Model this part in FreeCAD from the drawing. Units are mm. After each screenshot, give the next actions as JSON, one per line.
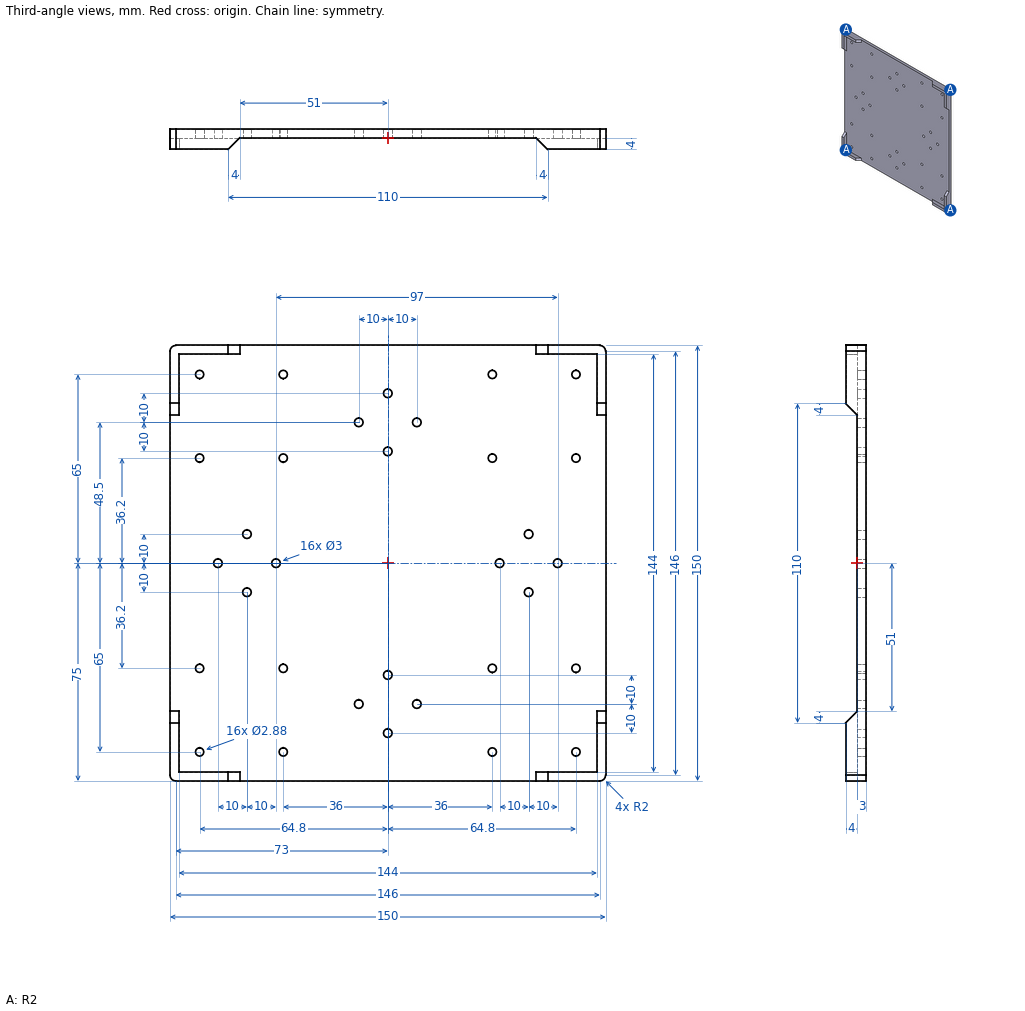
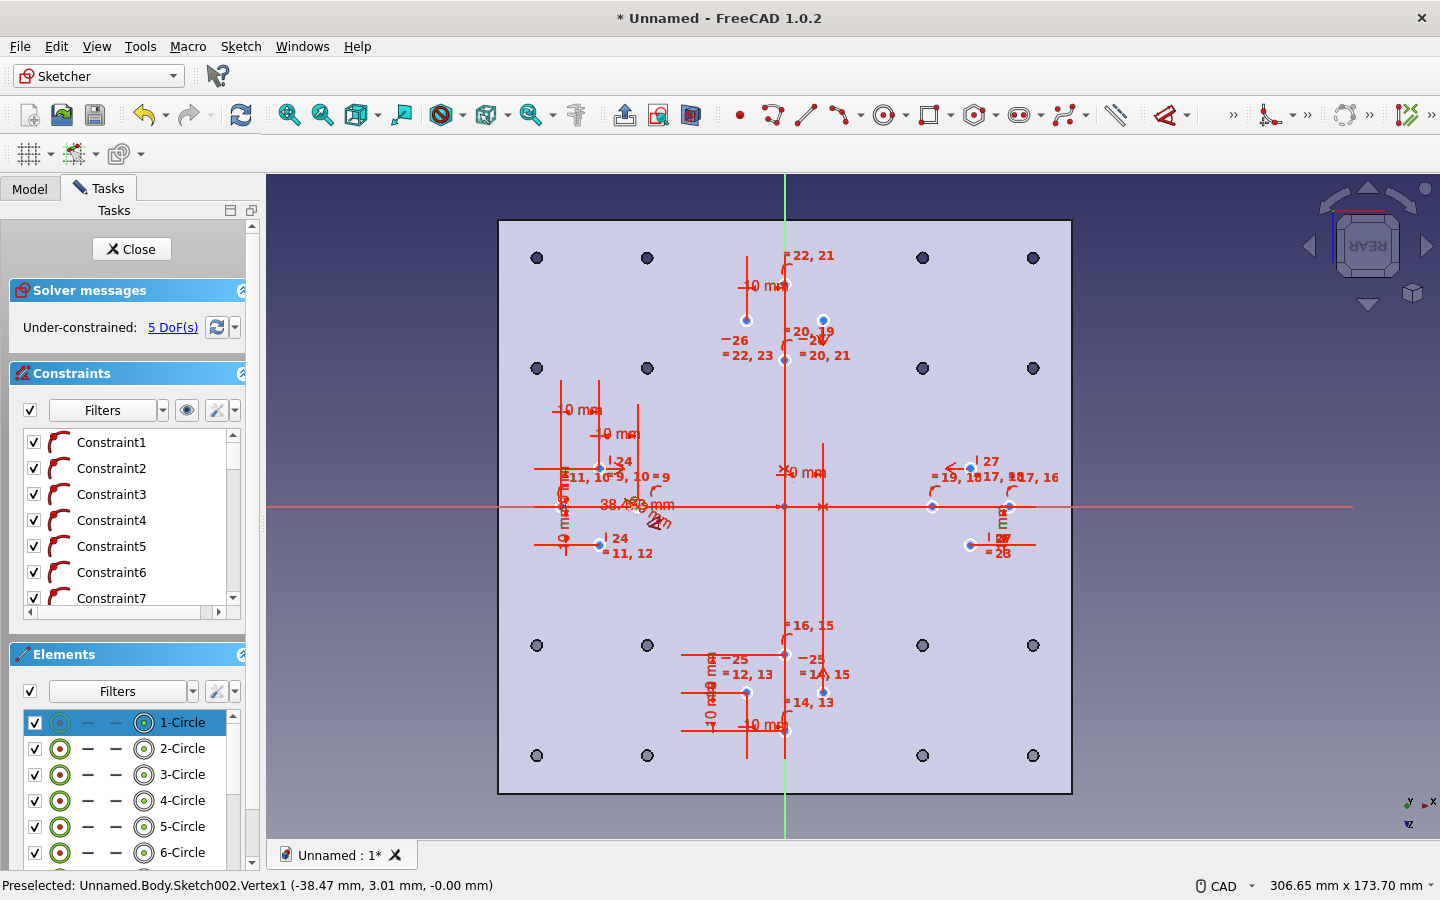
{"action": "left_click", "coordinate": [1009, 507]}
{"action": "left_click", "coordinate": [823, 541]}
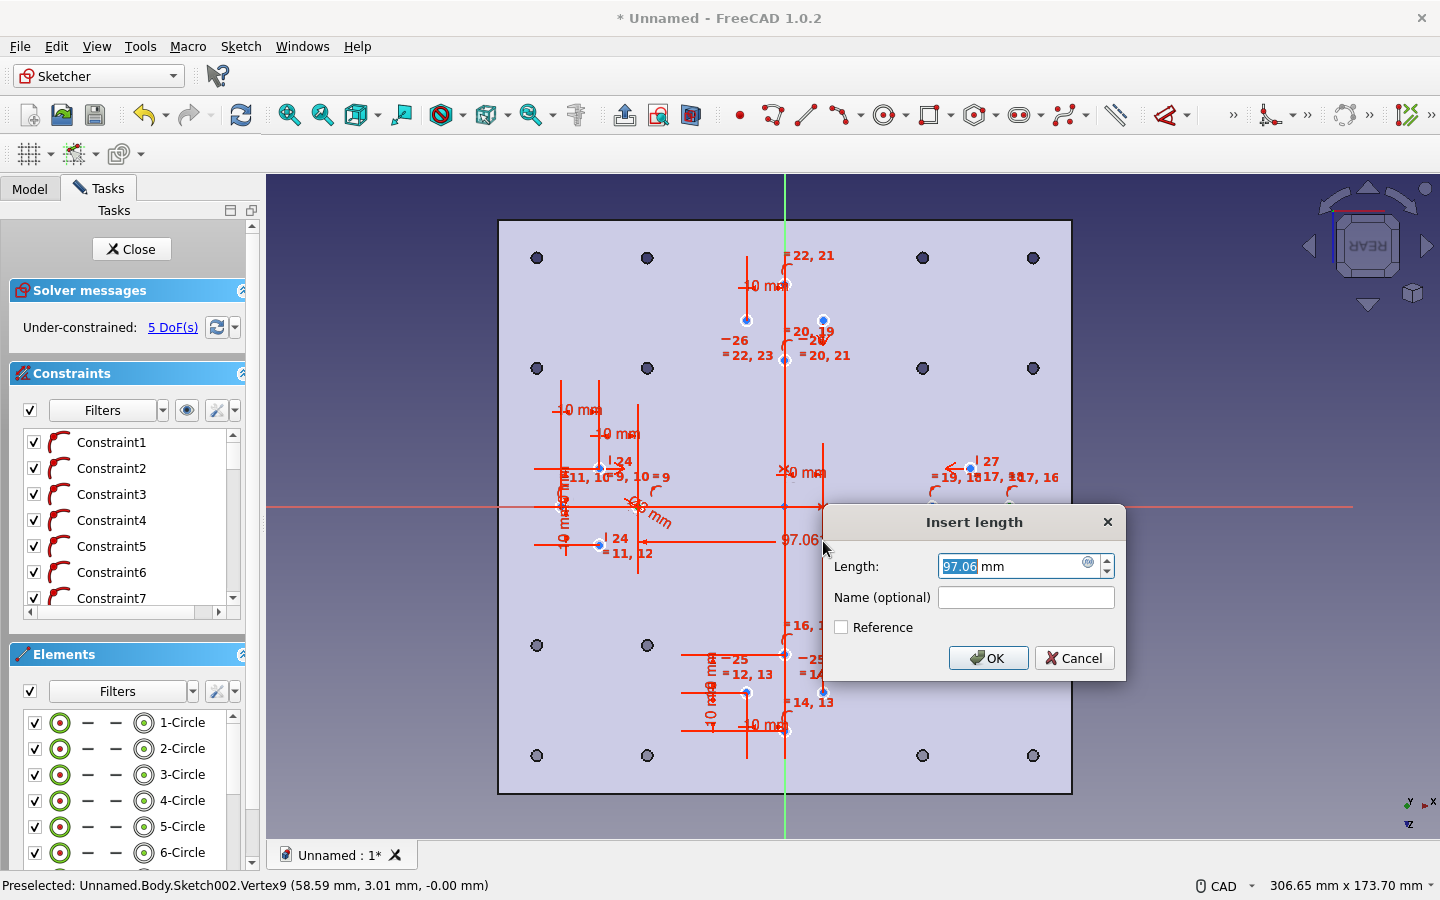
{"action": "type", "text": "97"}
{"action": "key", "text": "Return"}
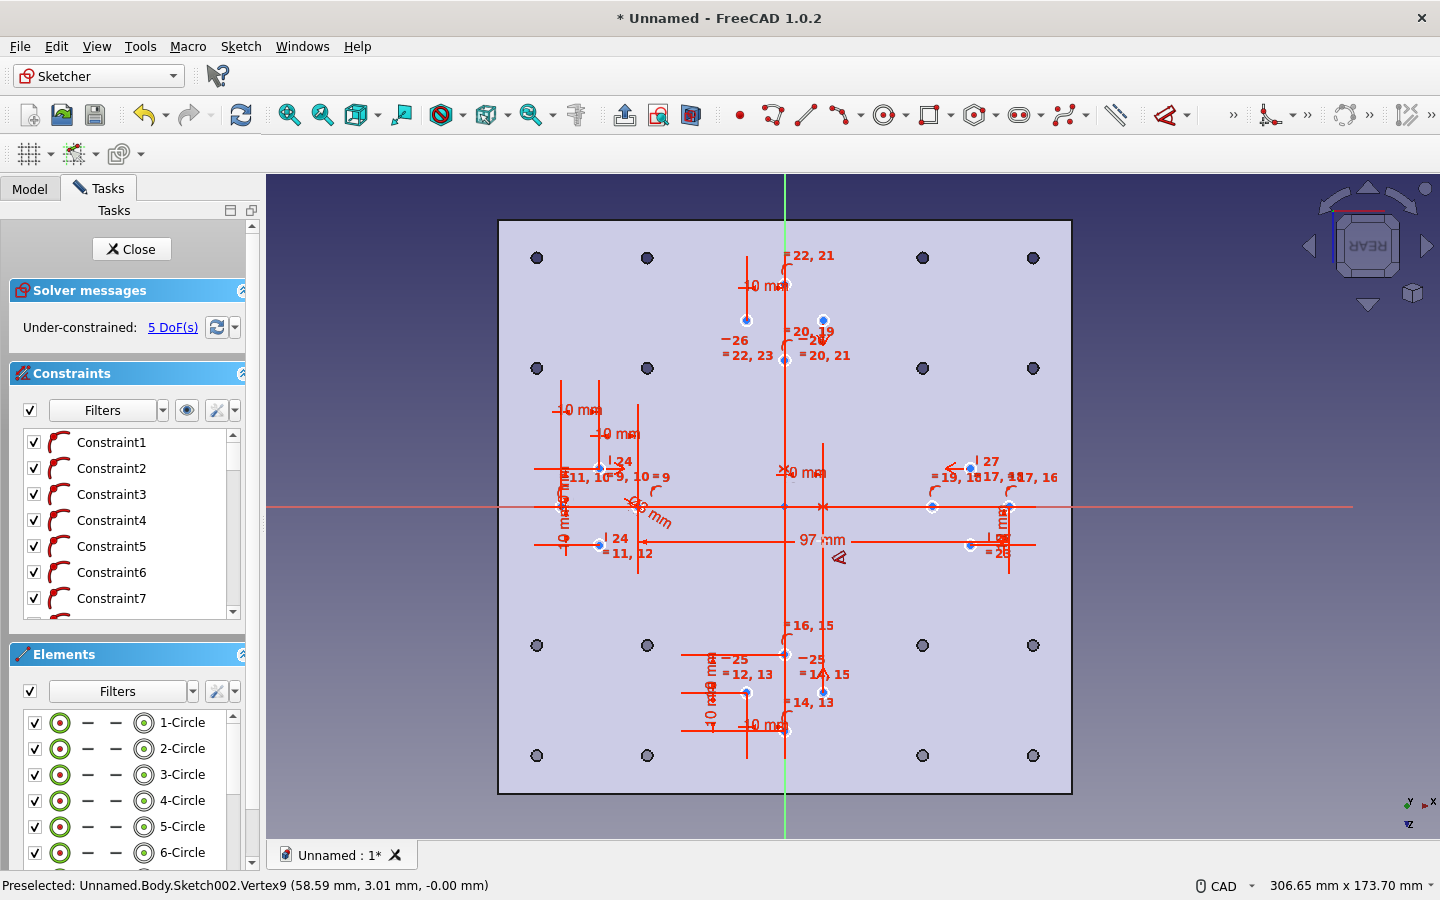
{"action": "left_click", "coordinate": [1009, 507]}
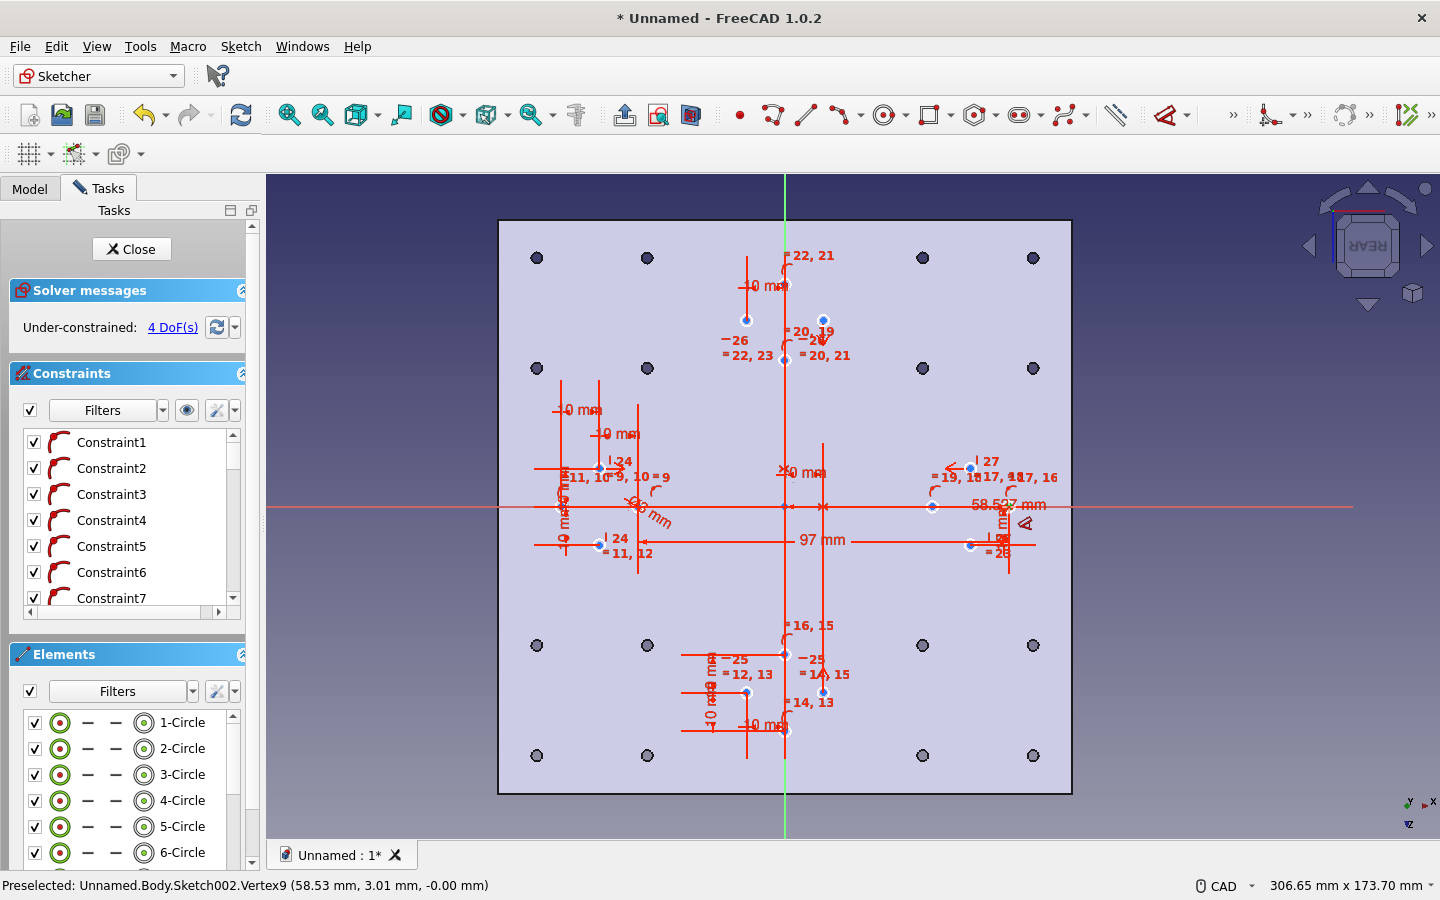
{"action": "left_click", "coordinate": [971, 469]}
{"action": "left_click", "coordinate": [990, 435]}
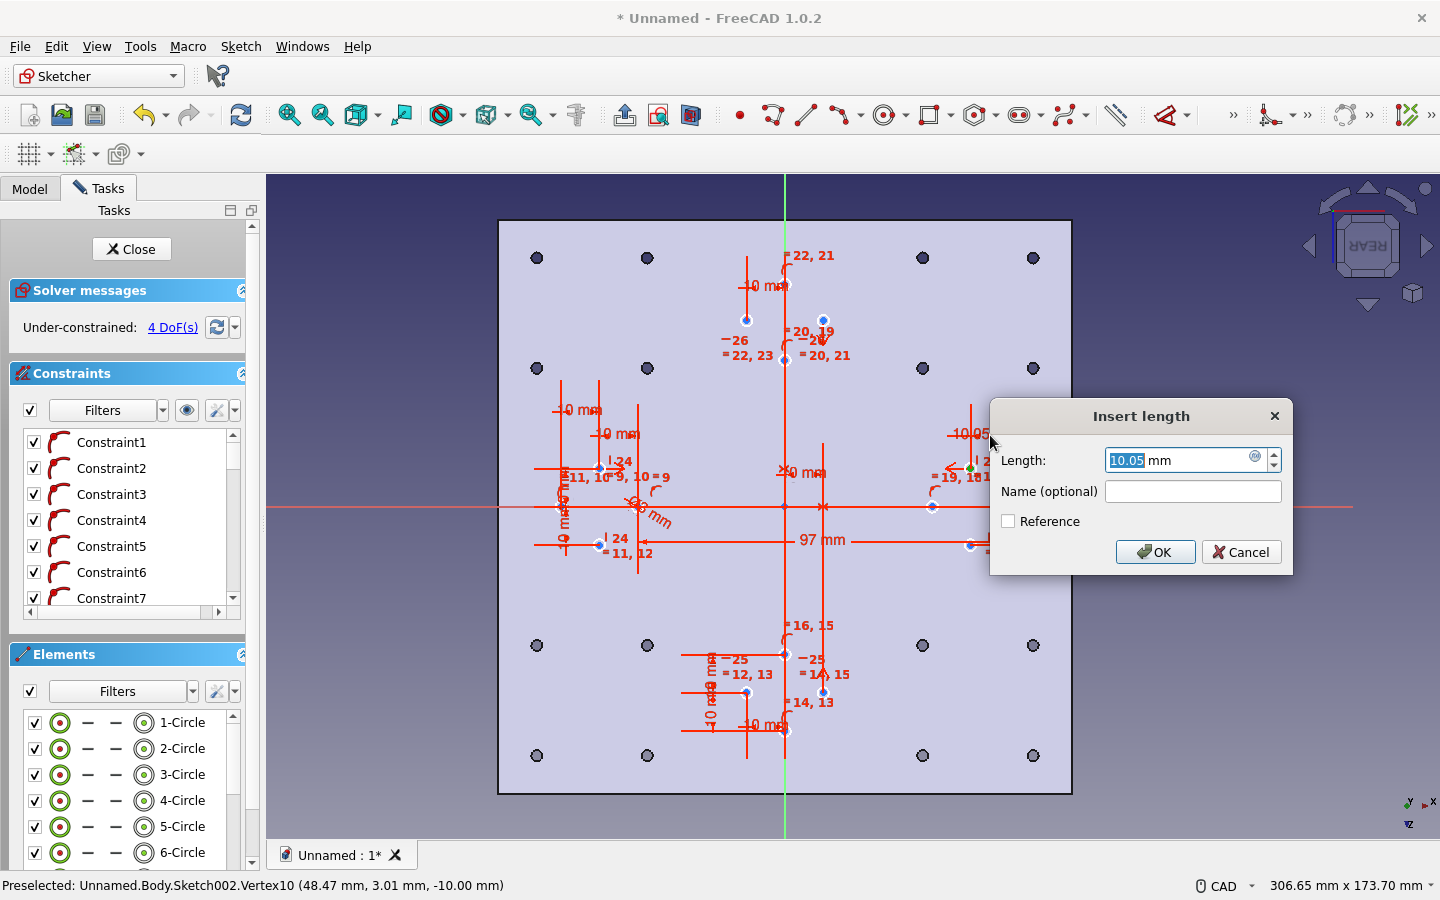
{"action": "type", "text": "10"}
{"action": "key", "text": "Return"}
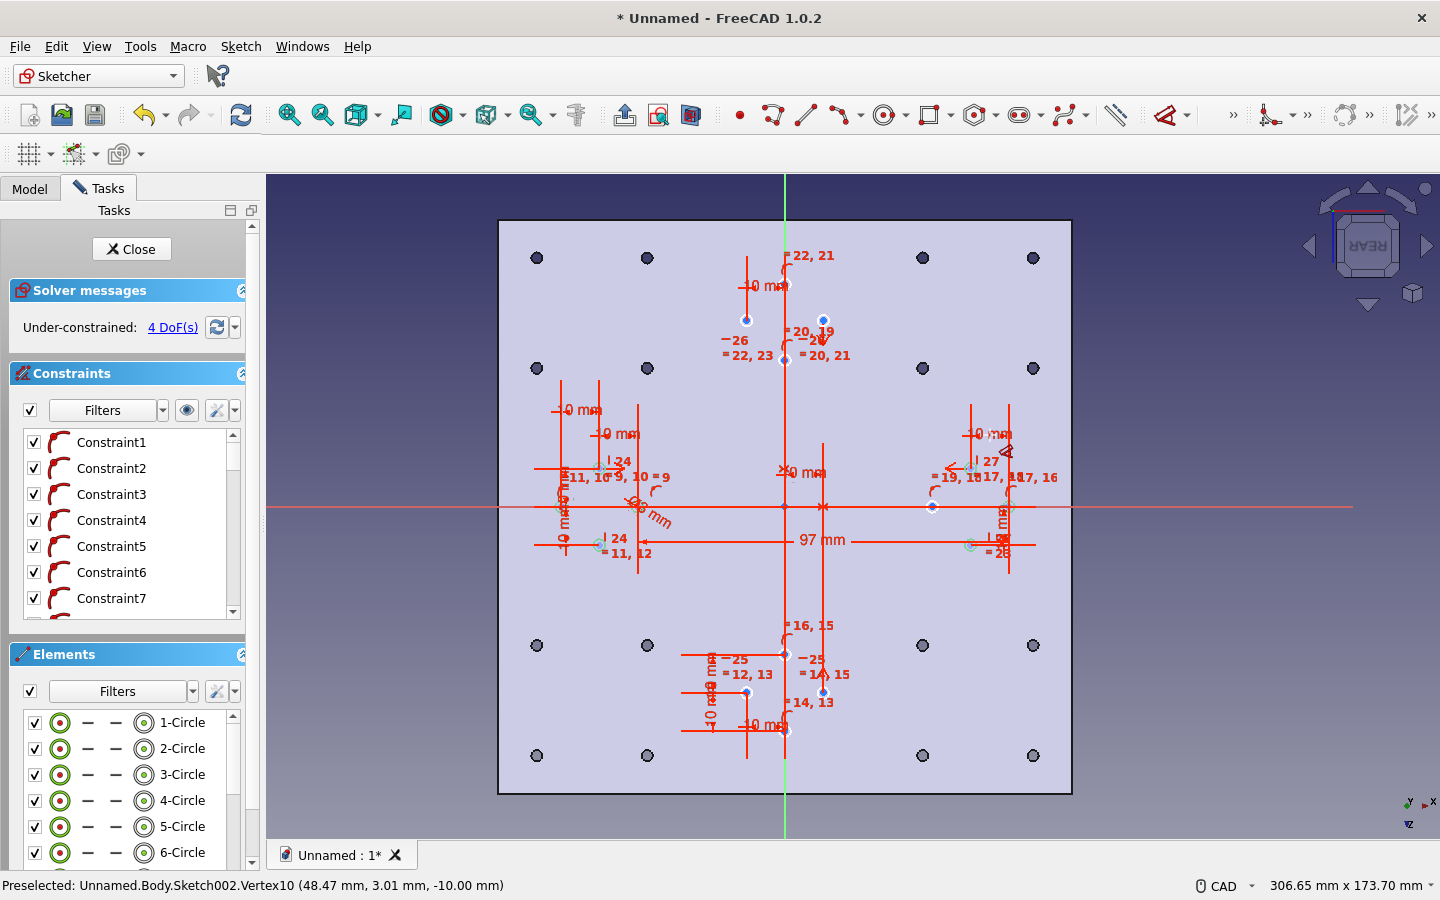
{"action": "left_click", "coordinate": [971, 469]}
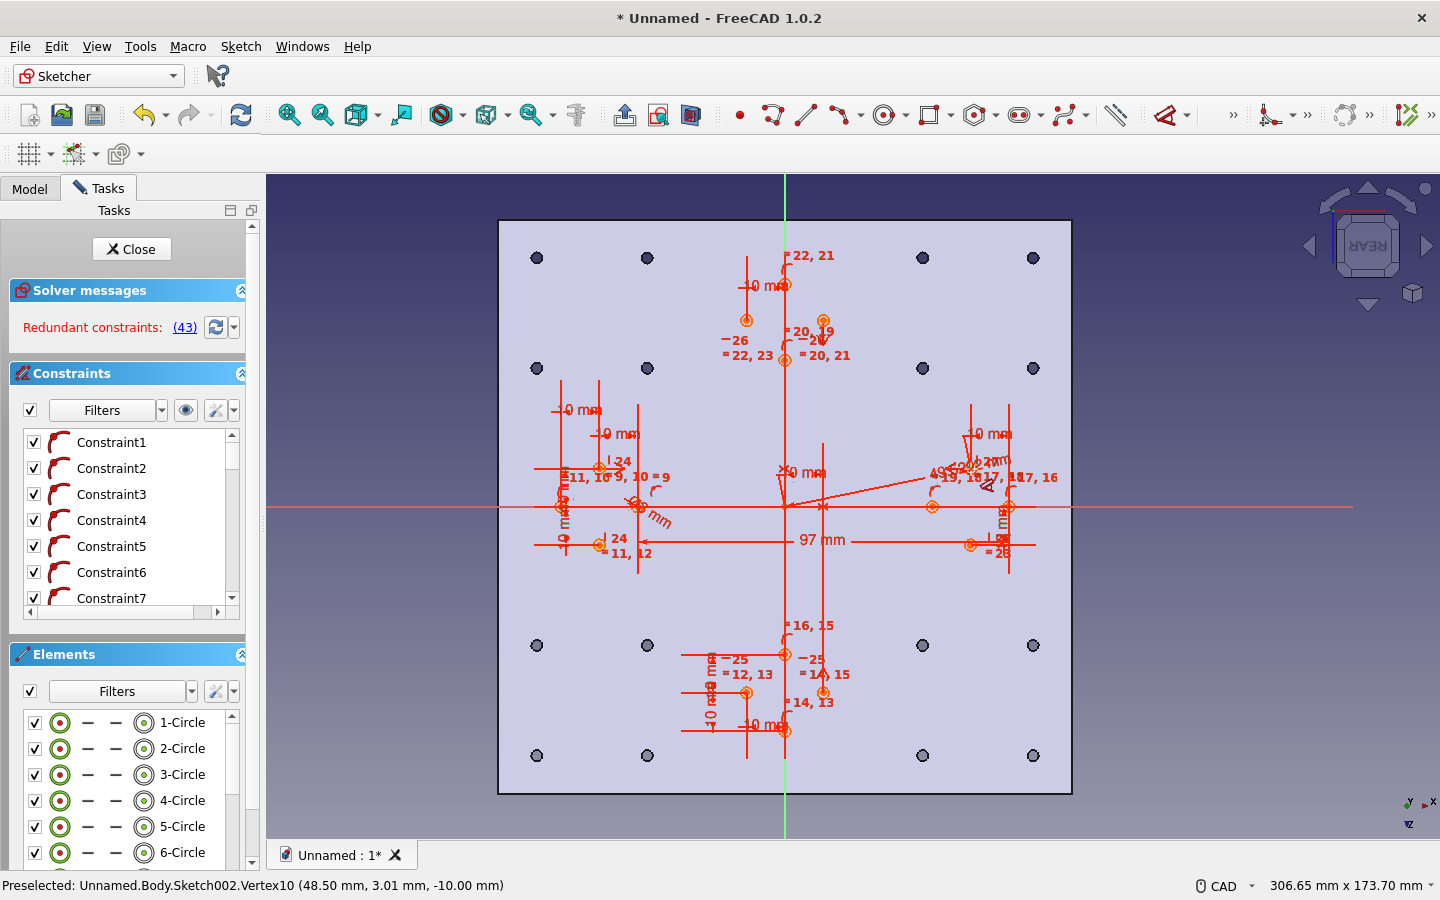
{"action": "left_click", "coordinate": [932, 507]}
{"action": "left_click", "coordinate": [951, 411]}